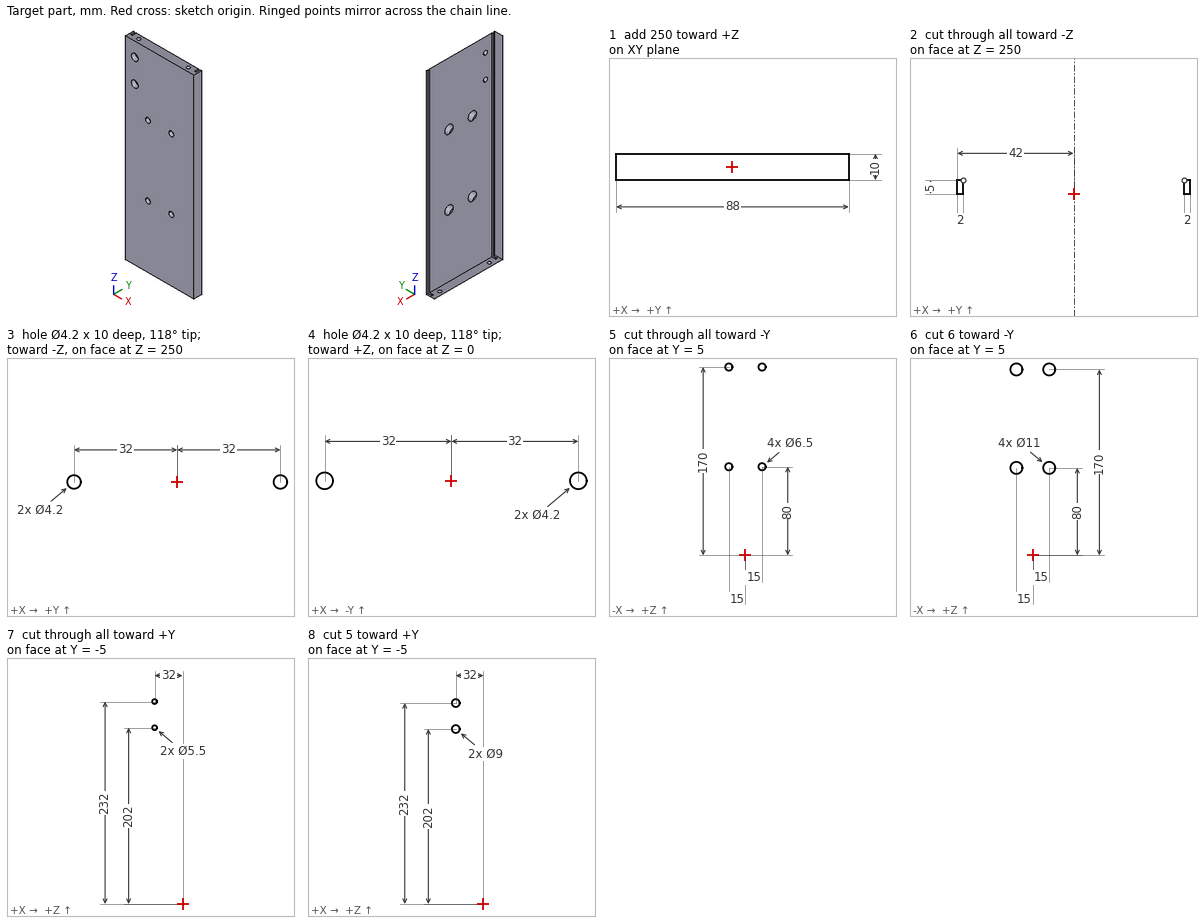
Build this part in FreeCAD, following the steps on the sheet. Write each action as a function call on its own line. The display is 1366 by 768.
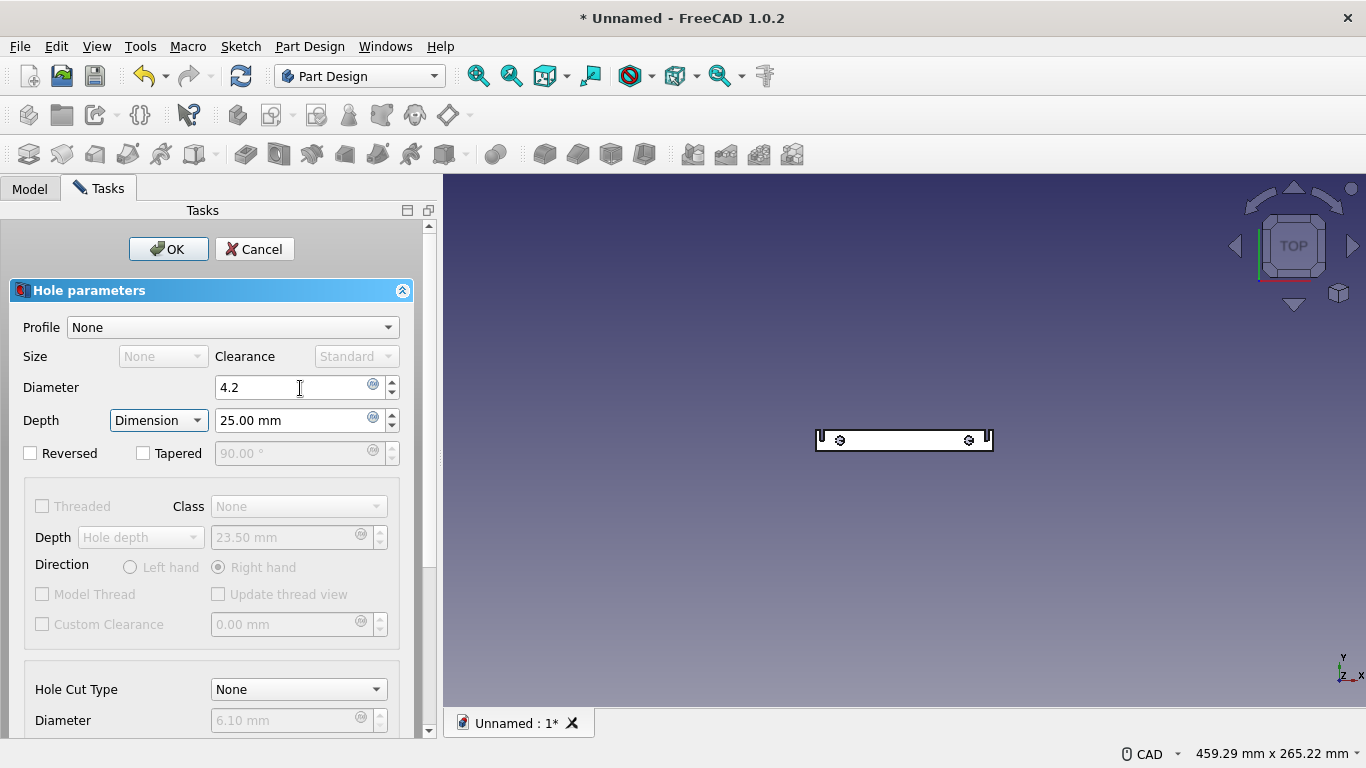
triple_click(300, 420)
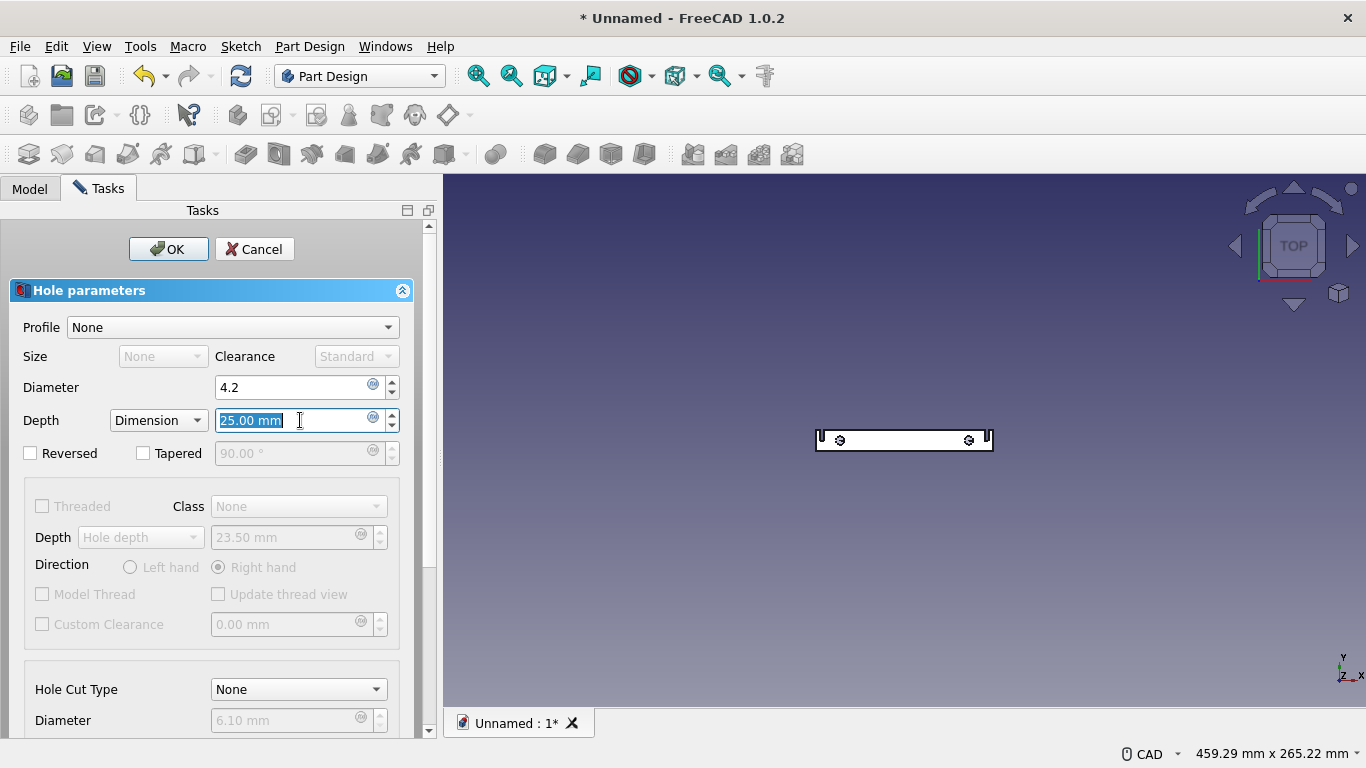
text(10)
key(Tab)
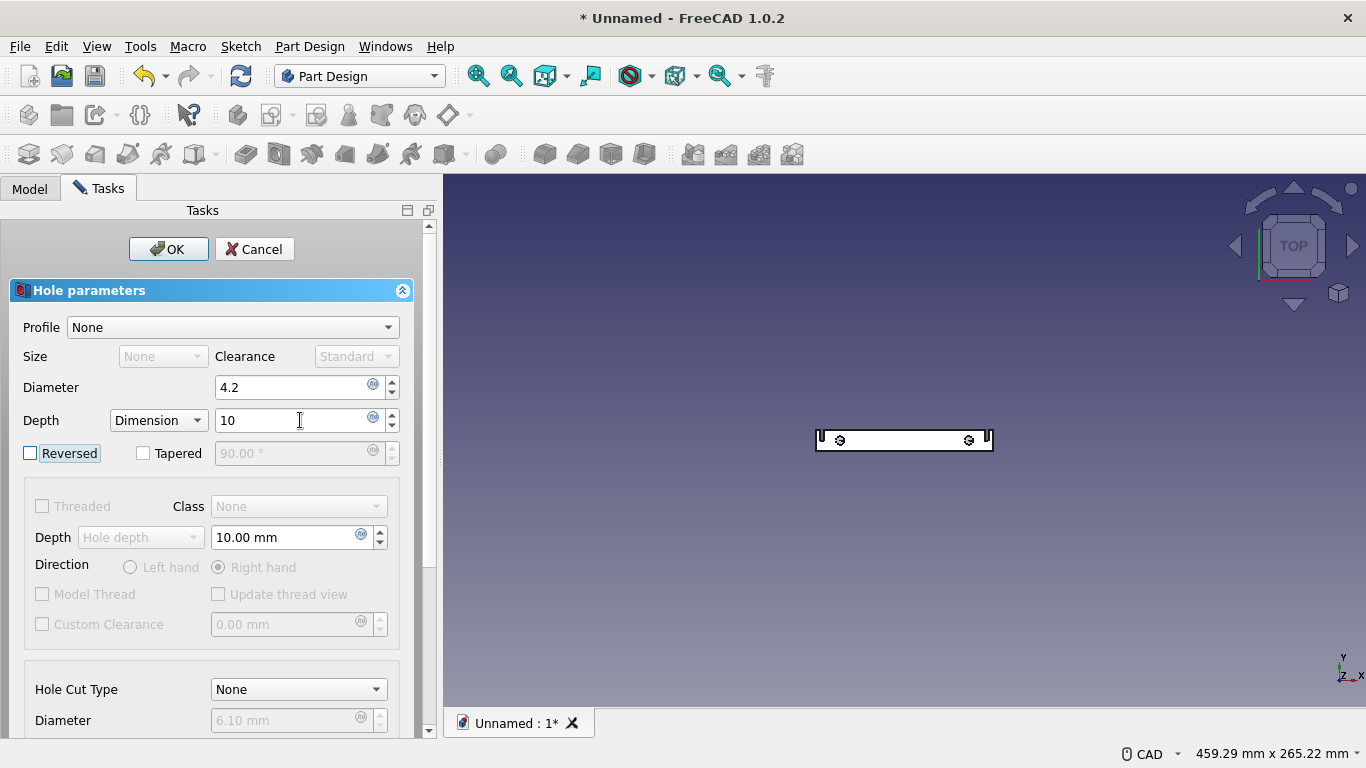
click(169, 249)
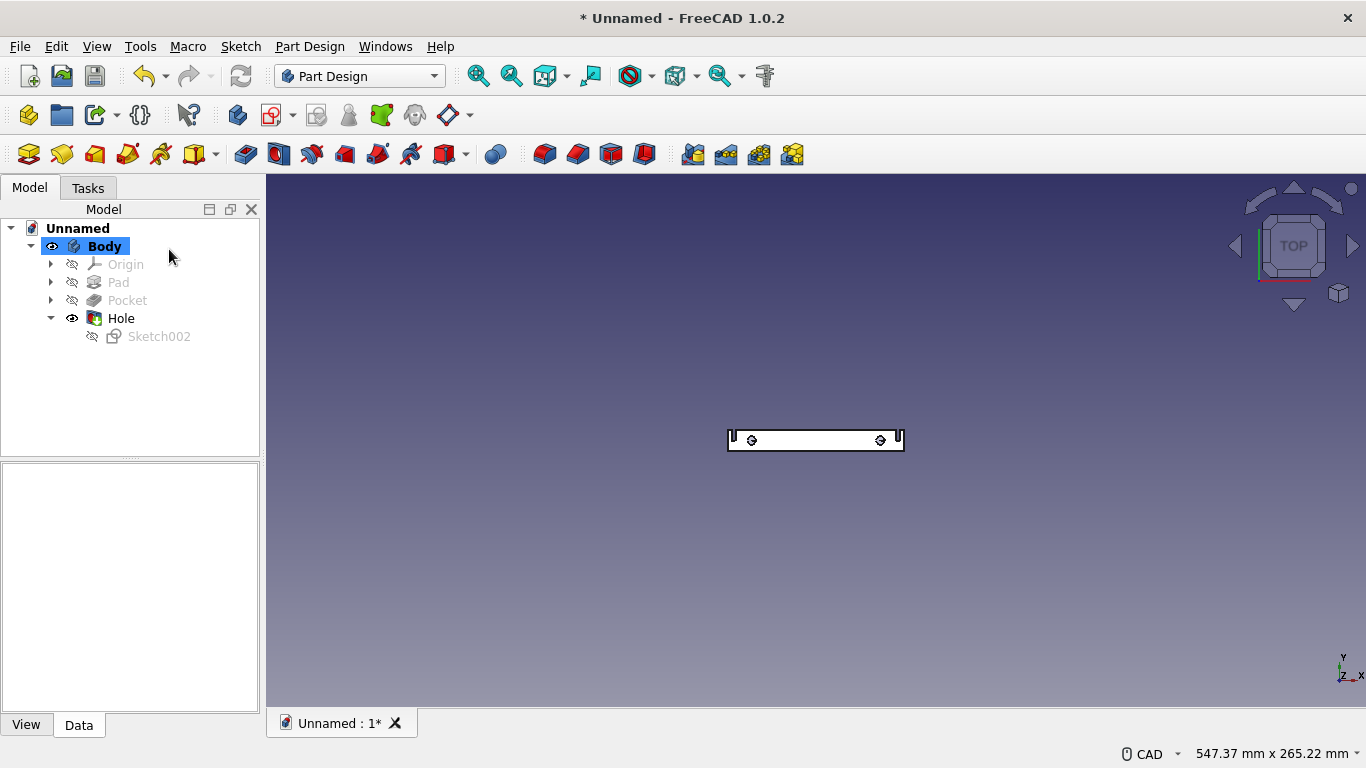
click(479, 76)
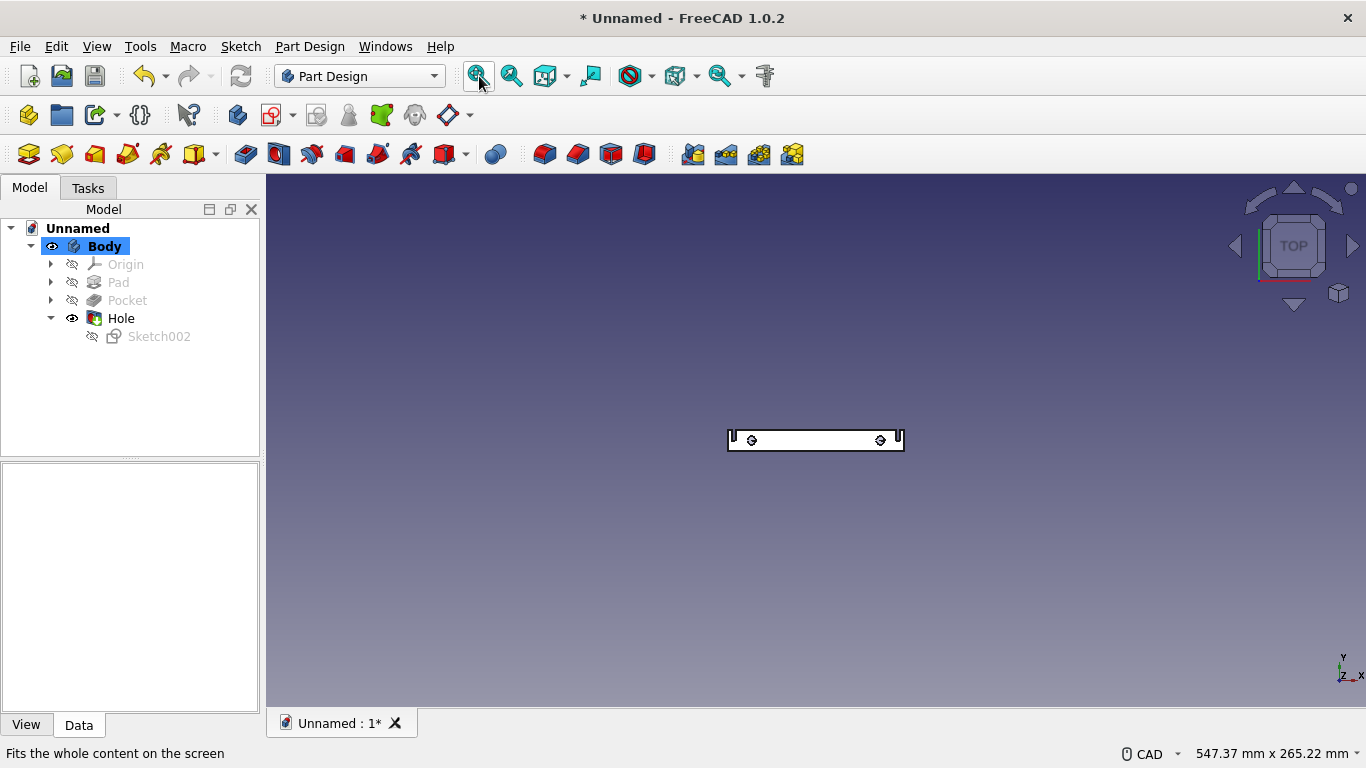
key(5)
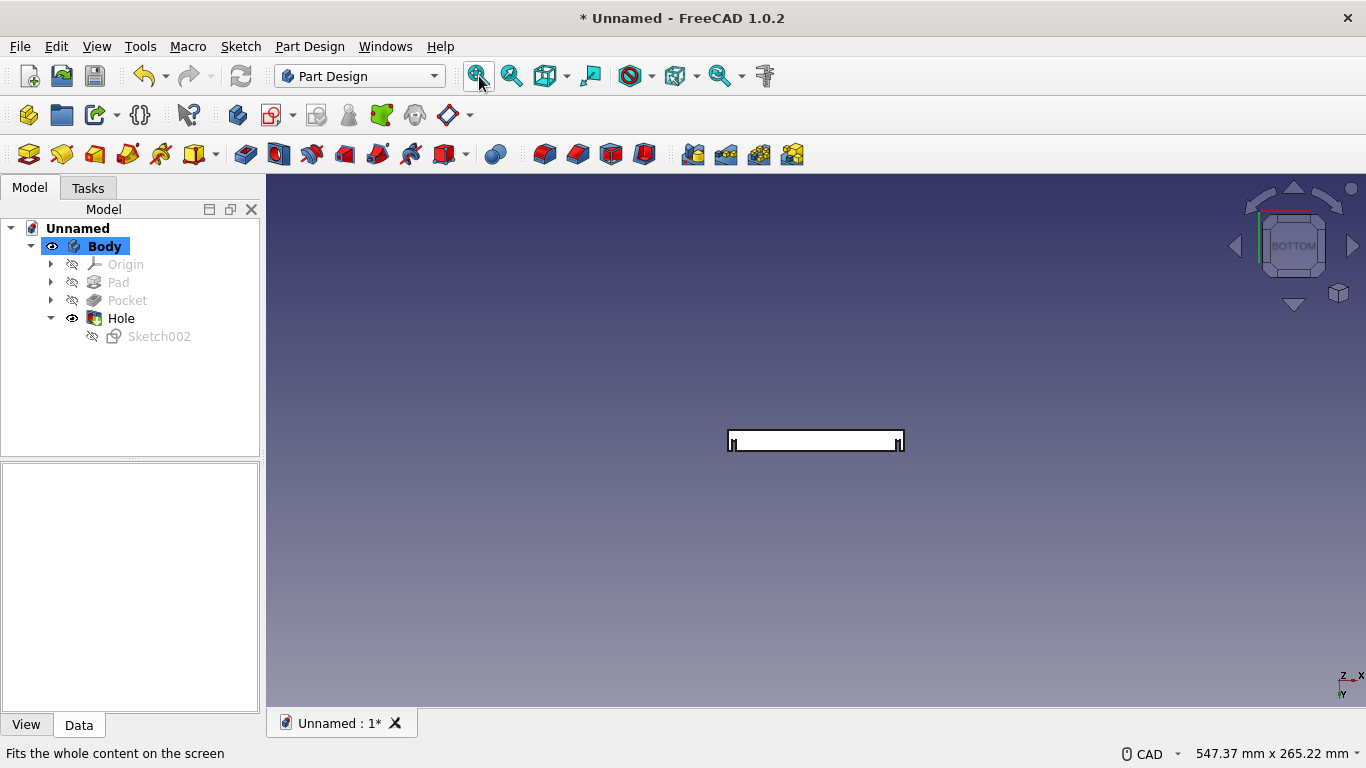
click(479, 76)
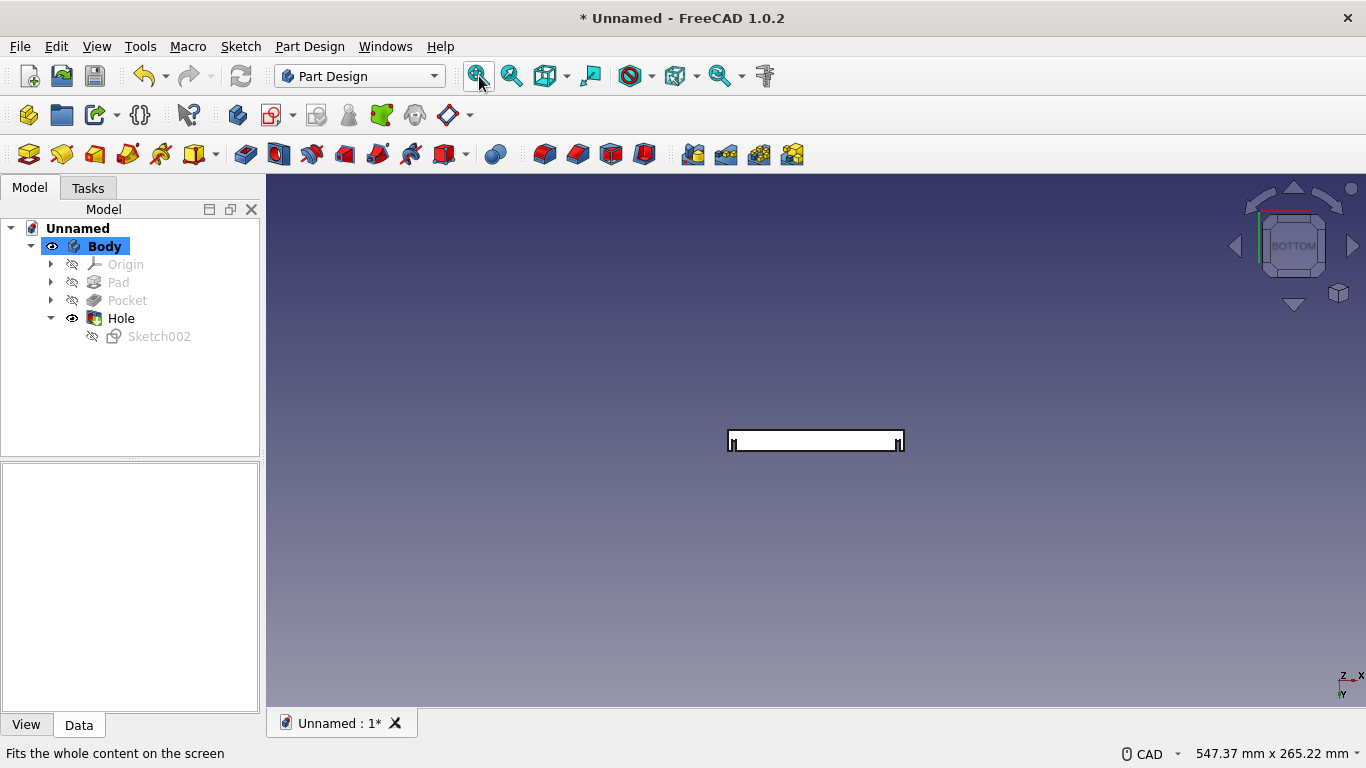
click(867, 439)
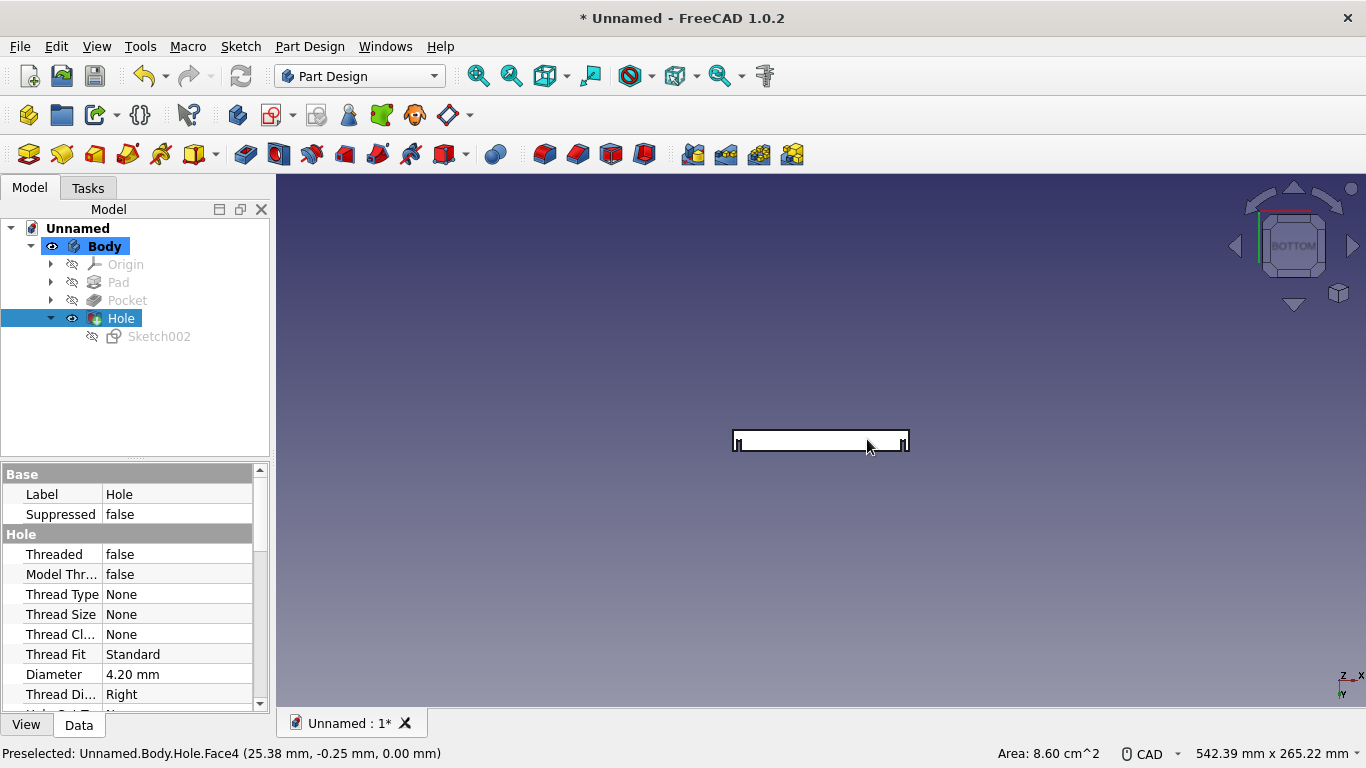
click(270, 116)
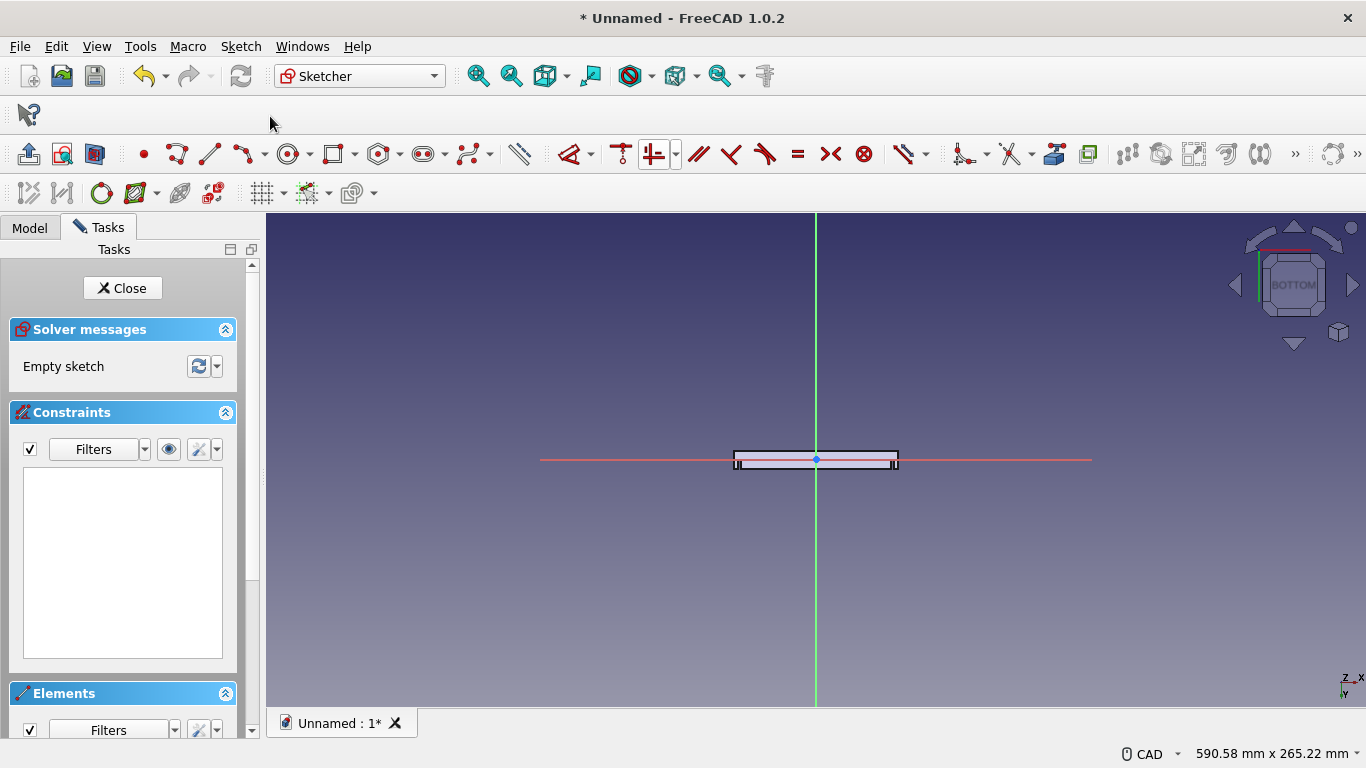
scroll(833, 460, up, 8)